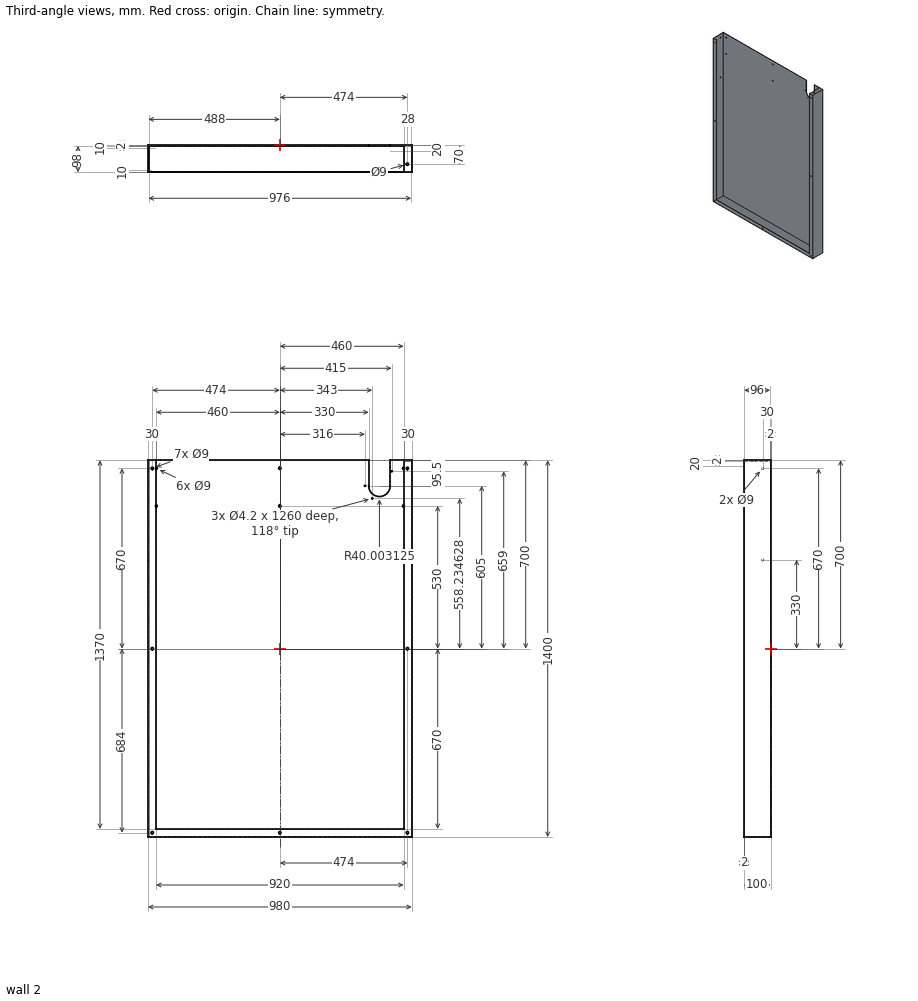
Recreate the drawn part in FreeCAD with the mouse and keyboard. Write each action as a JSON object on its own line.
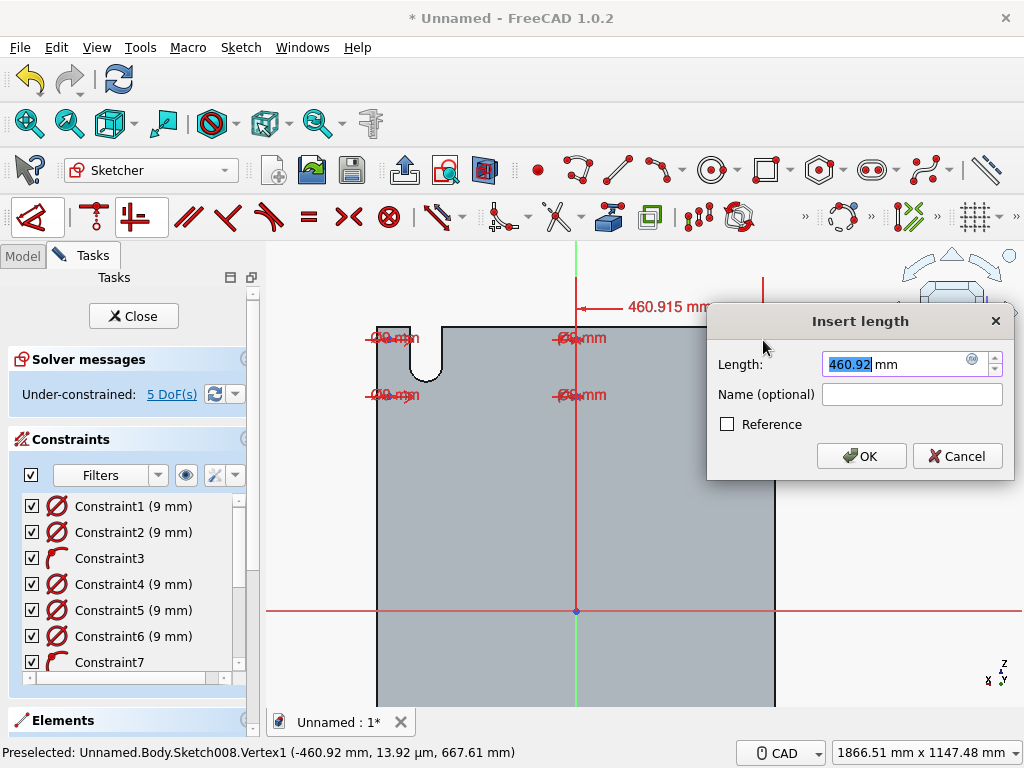
{"action": "type", "text": "460"}
{"action": "key", "text": "Return"}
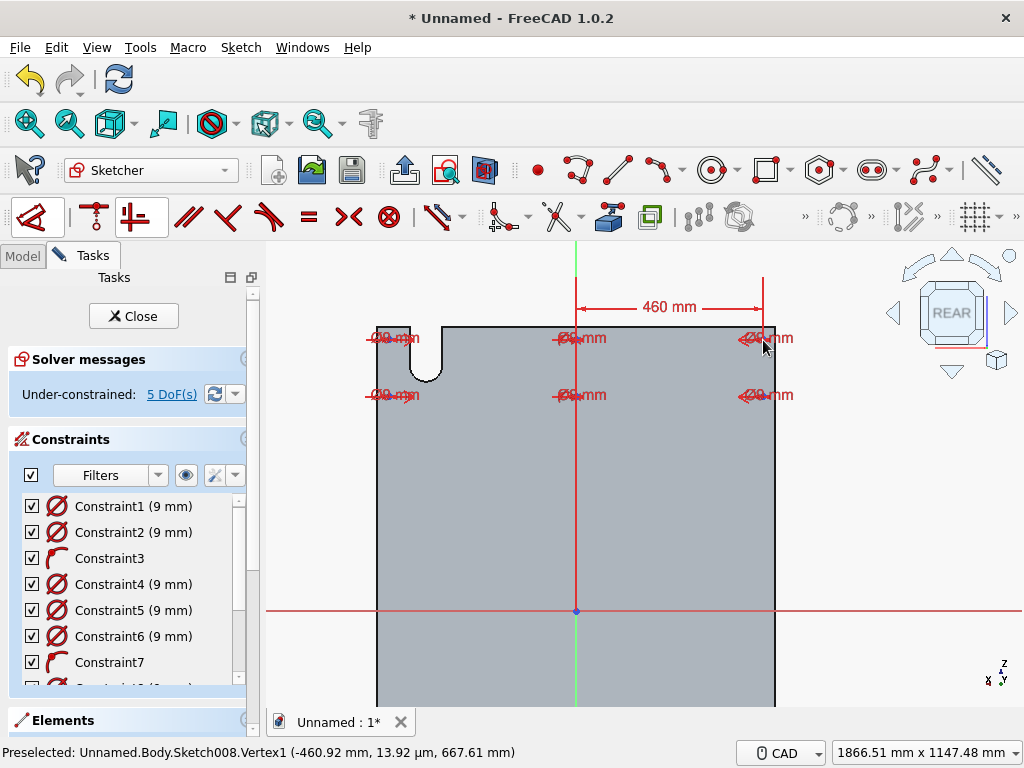
{"action": "left_click", "coordinate": [763, 340]}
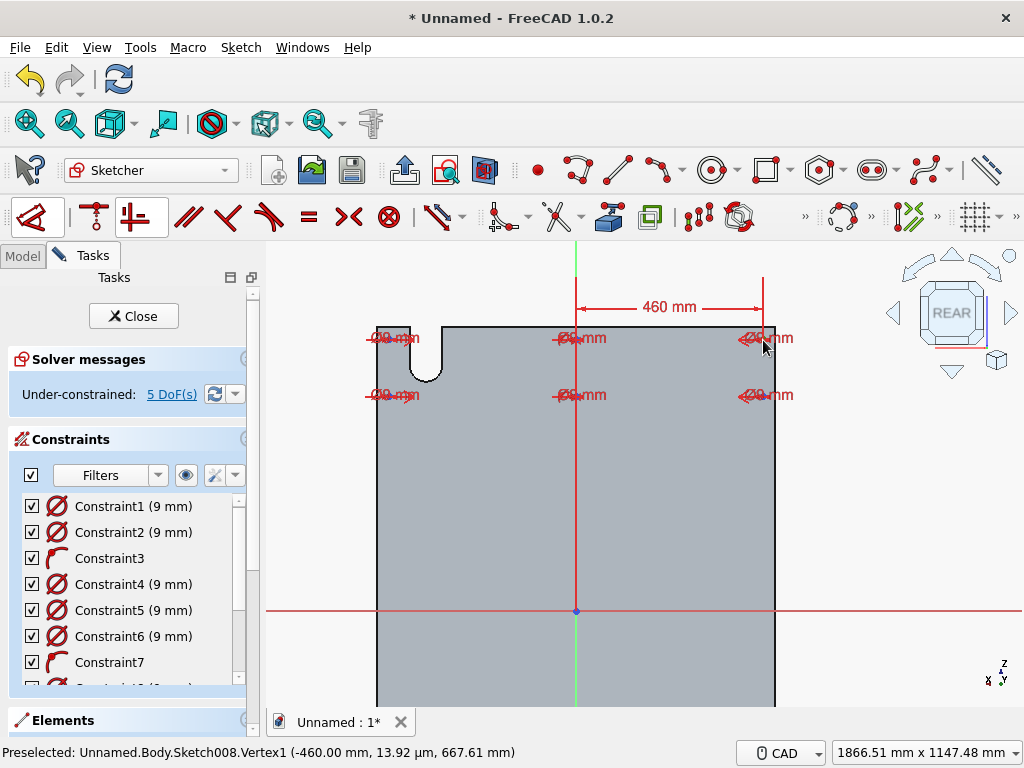
{"action": "left_click", "coordinate": [58, 218]}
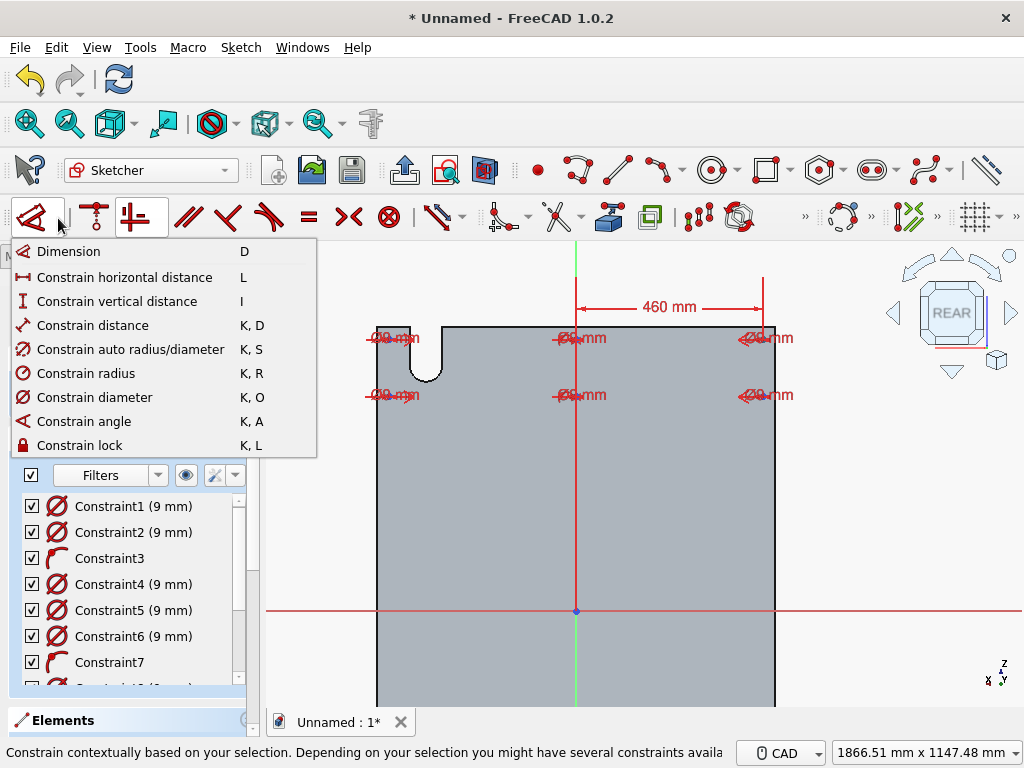
{"action": "left_click", "coordinate": [164, 301]}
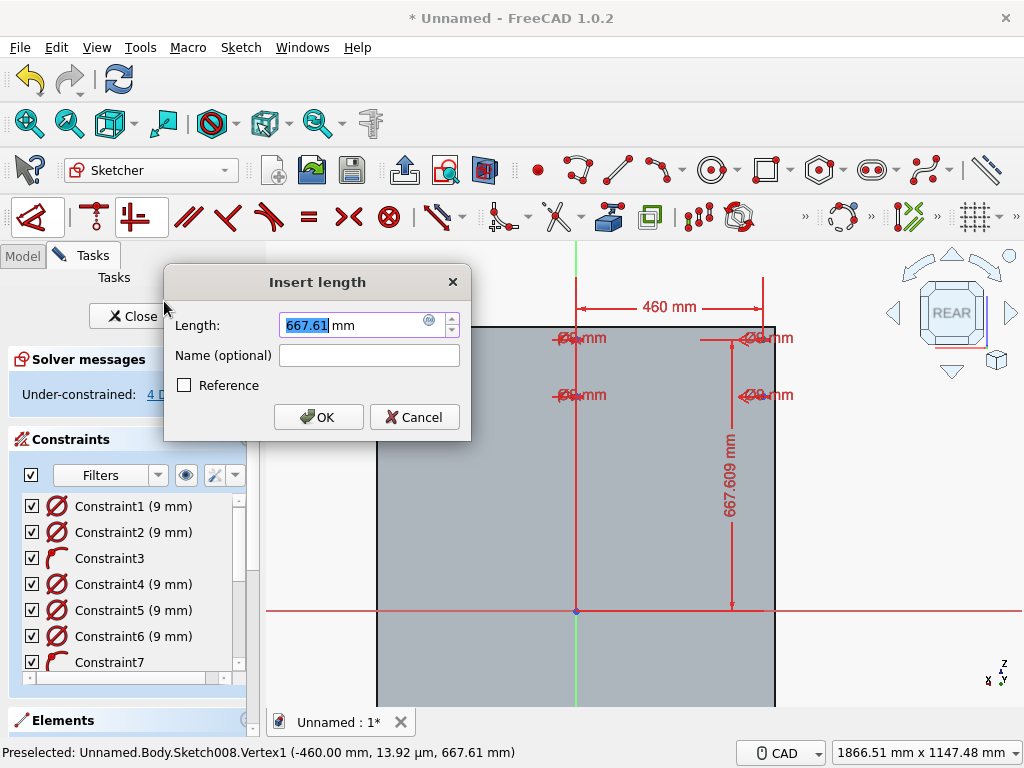
{"action": "type", "text": "670"}
{"action": "key", "text": "Return"}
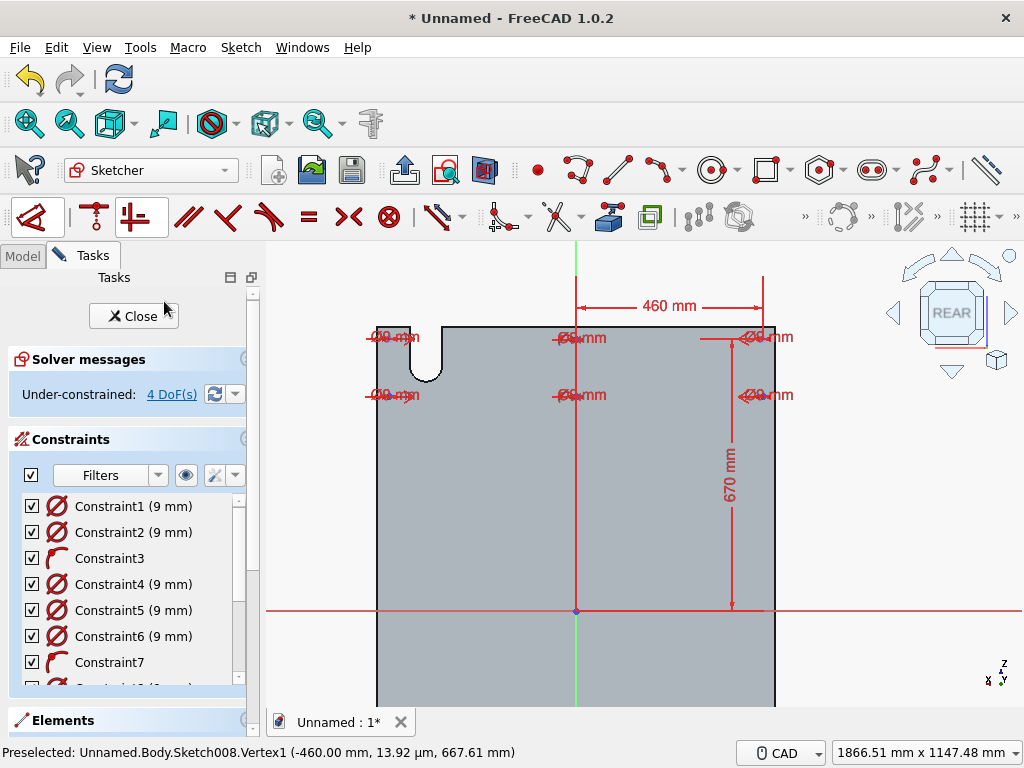
{"action": "left_click", "coordinate": [576, 397]}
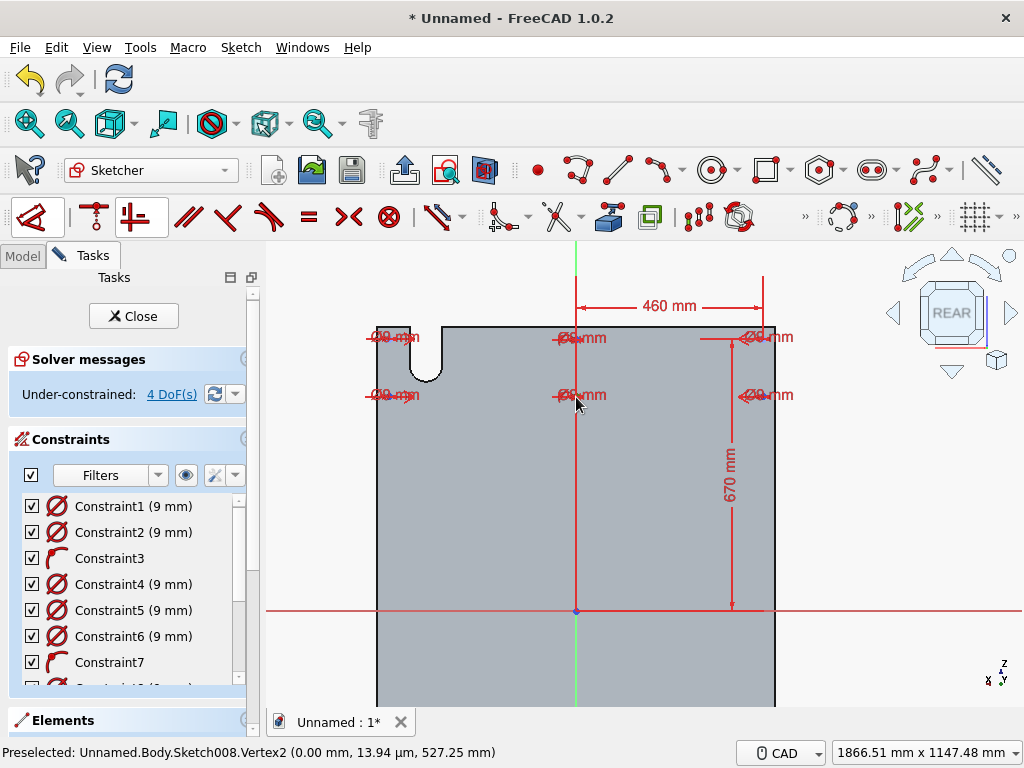
{"action": "left_click", "coordinate": [58, 218]}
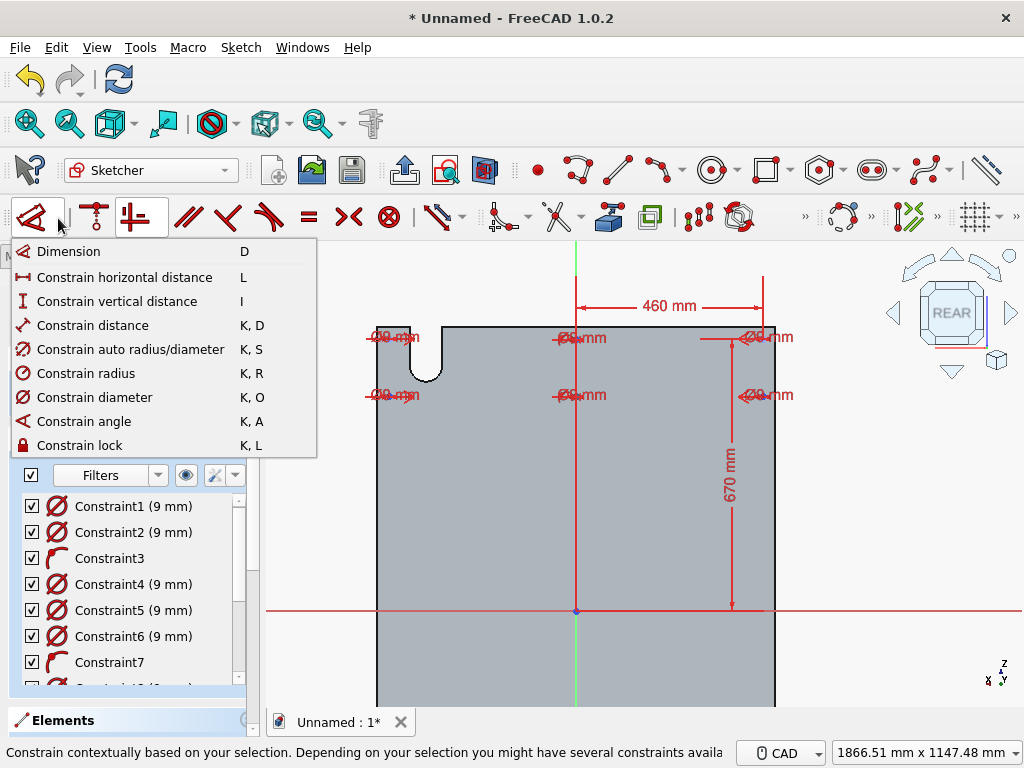
{"action": "left_click", "coordinate": [164, 301]}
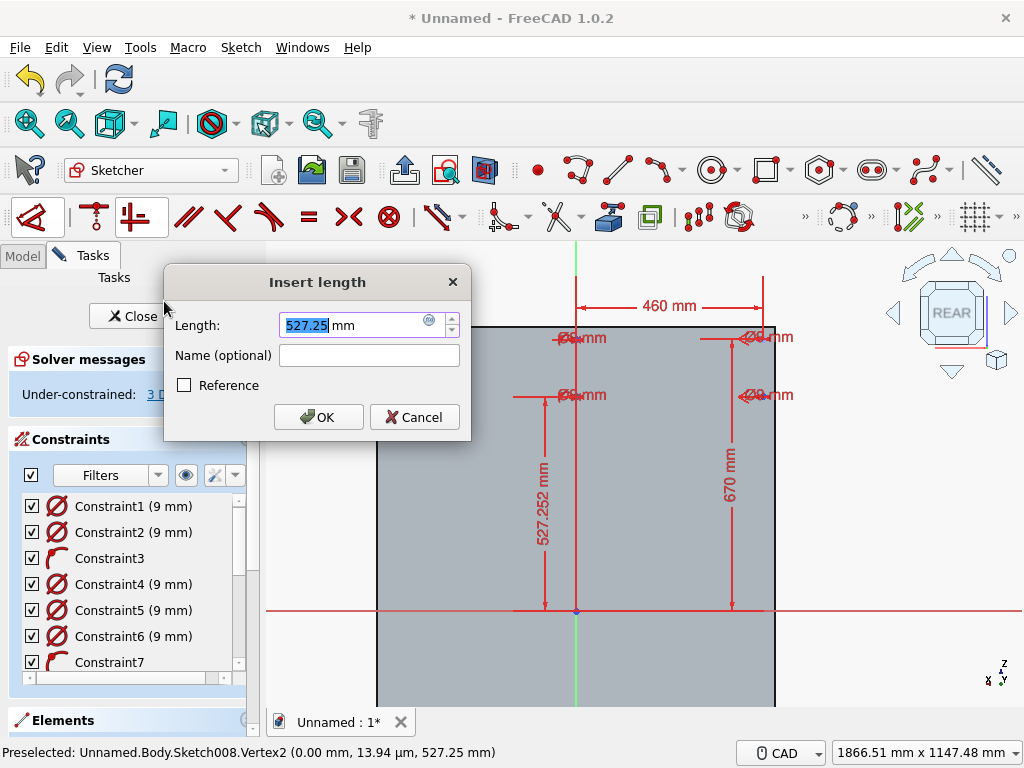
{"action": "type", "text": "530"}
{"action": "key", "text": "Return"}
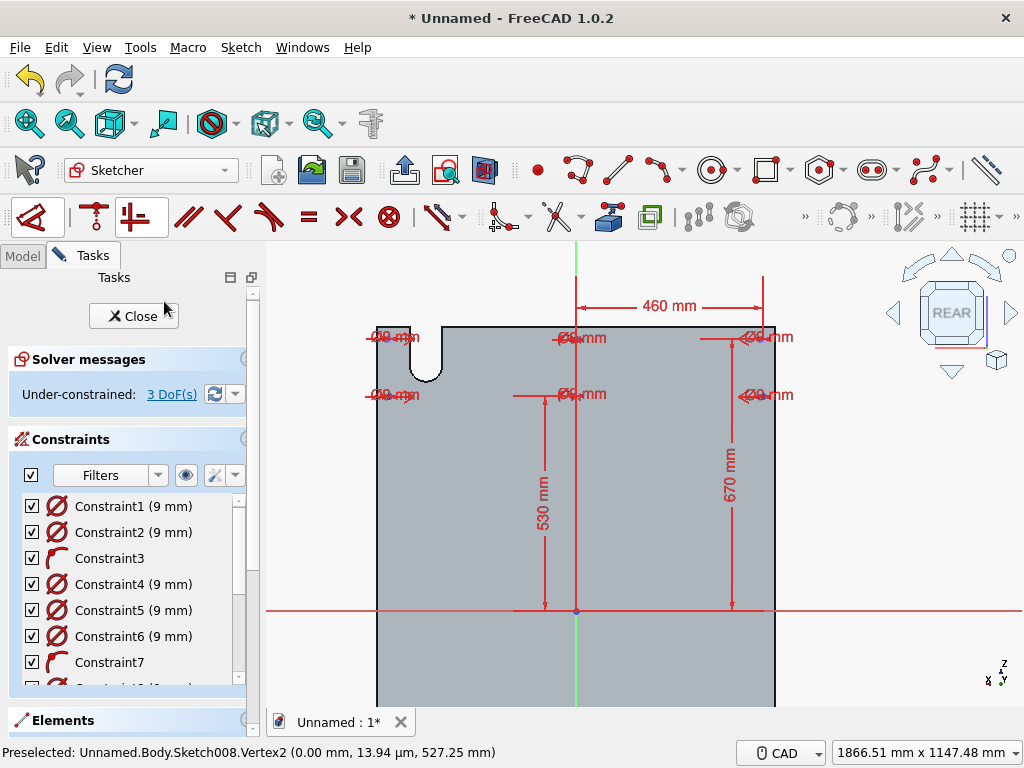
{"action": "left_click", "coordinate": [389, 397]}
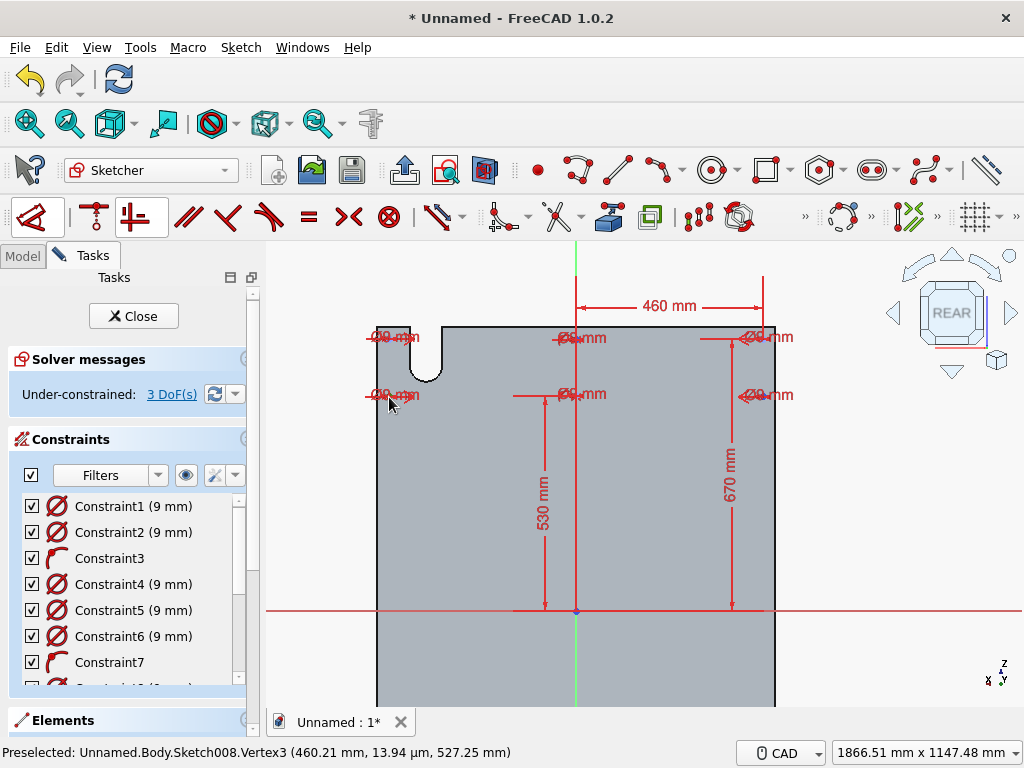
{"action": "key", "text": "l"}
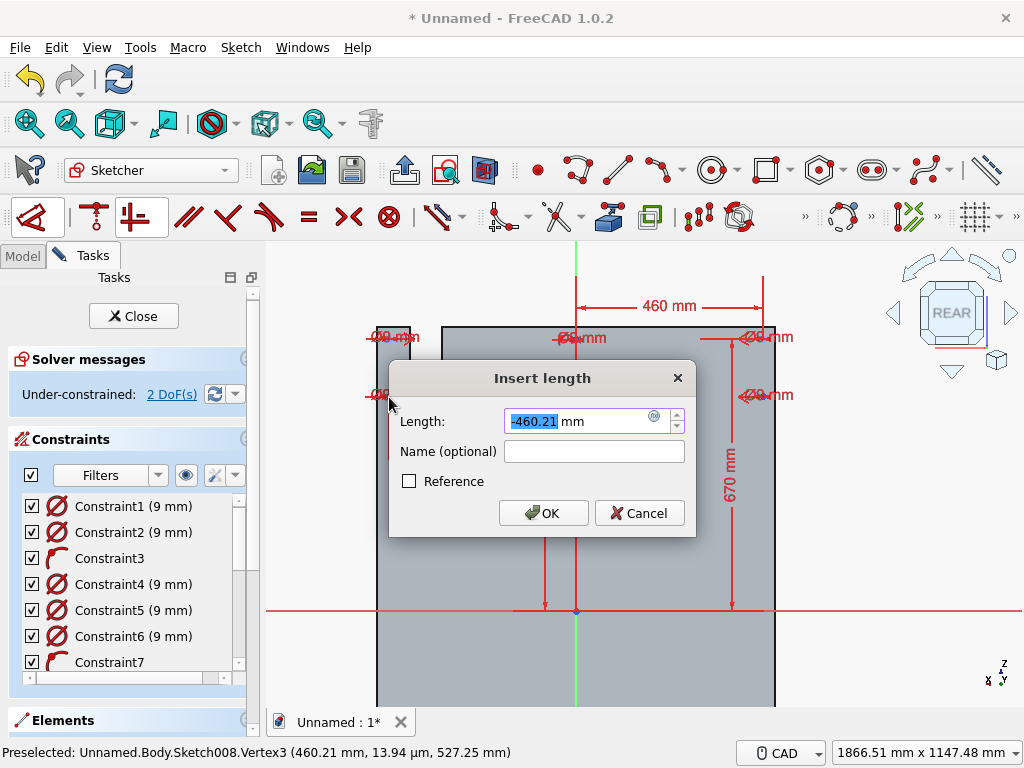
{"action": "type", "text": "-460"}
{"action": "key", "text": "Return"}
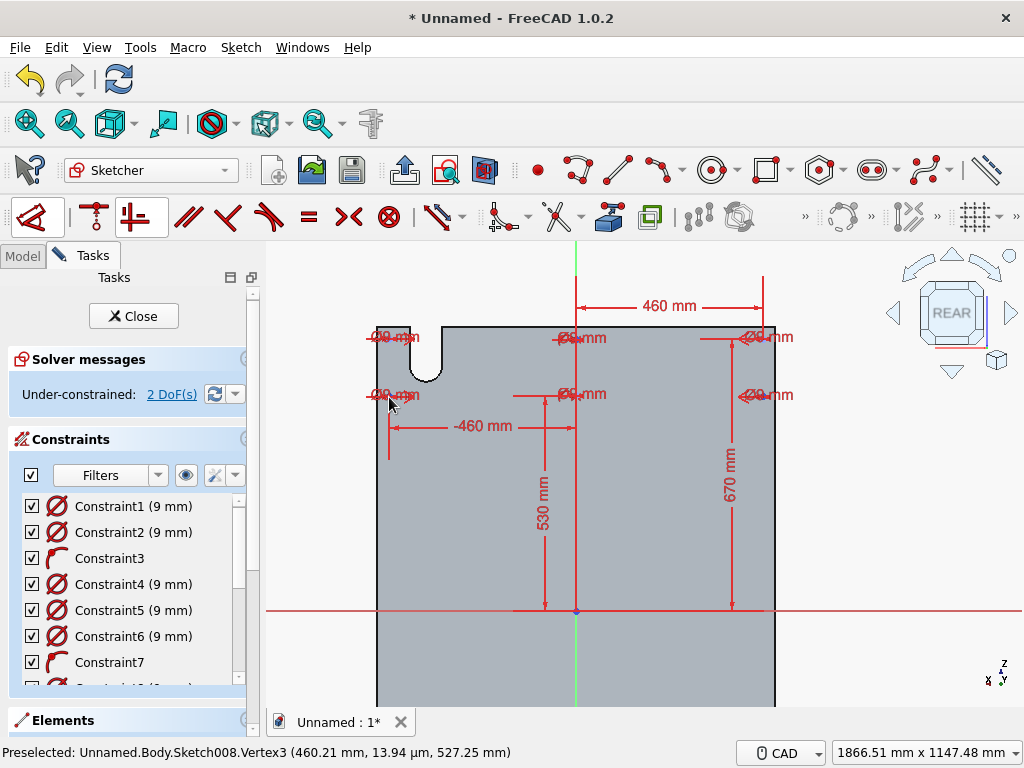
{"action": "left_click", "coordinate": [389, 397]}